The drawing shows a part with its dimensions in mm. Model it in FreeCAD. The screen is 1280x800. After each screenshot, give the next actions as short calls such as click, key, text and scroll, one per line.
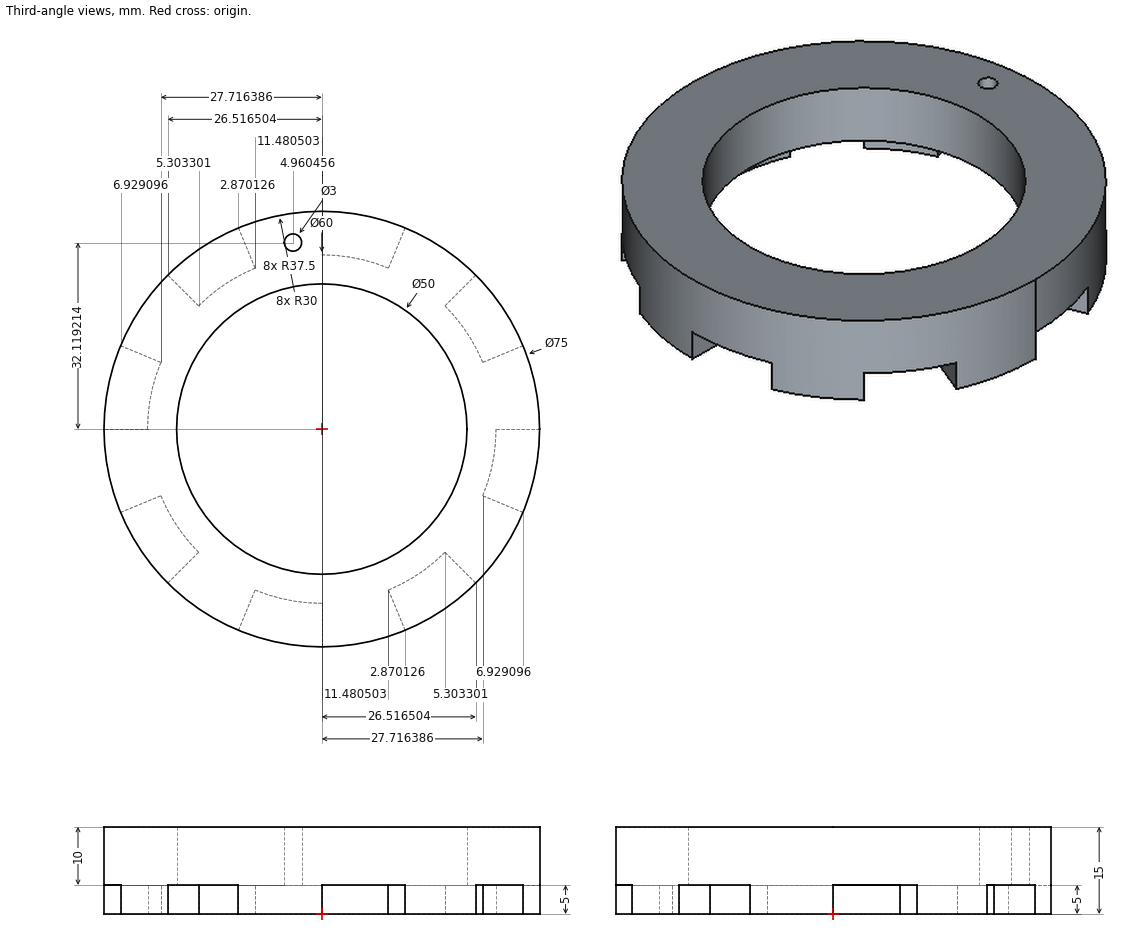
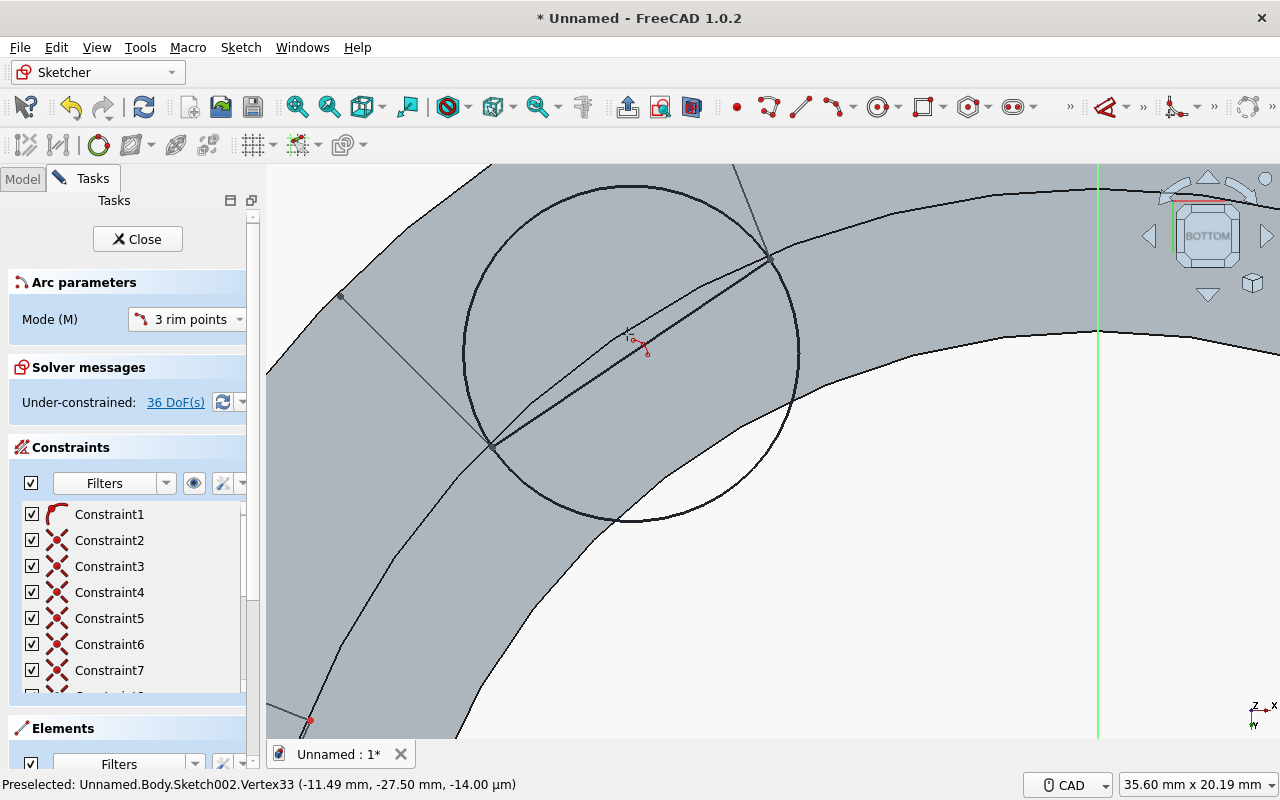
click(623, 333)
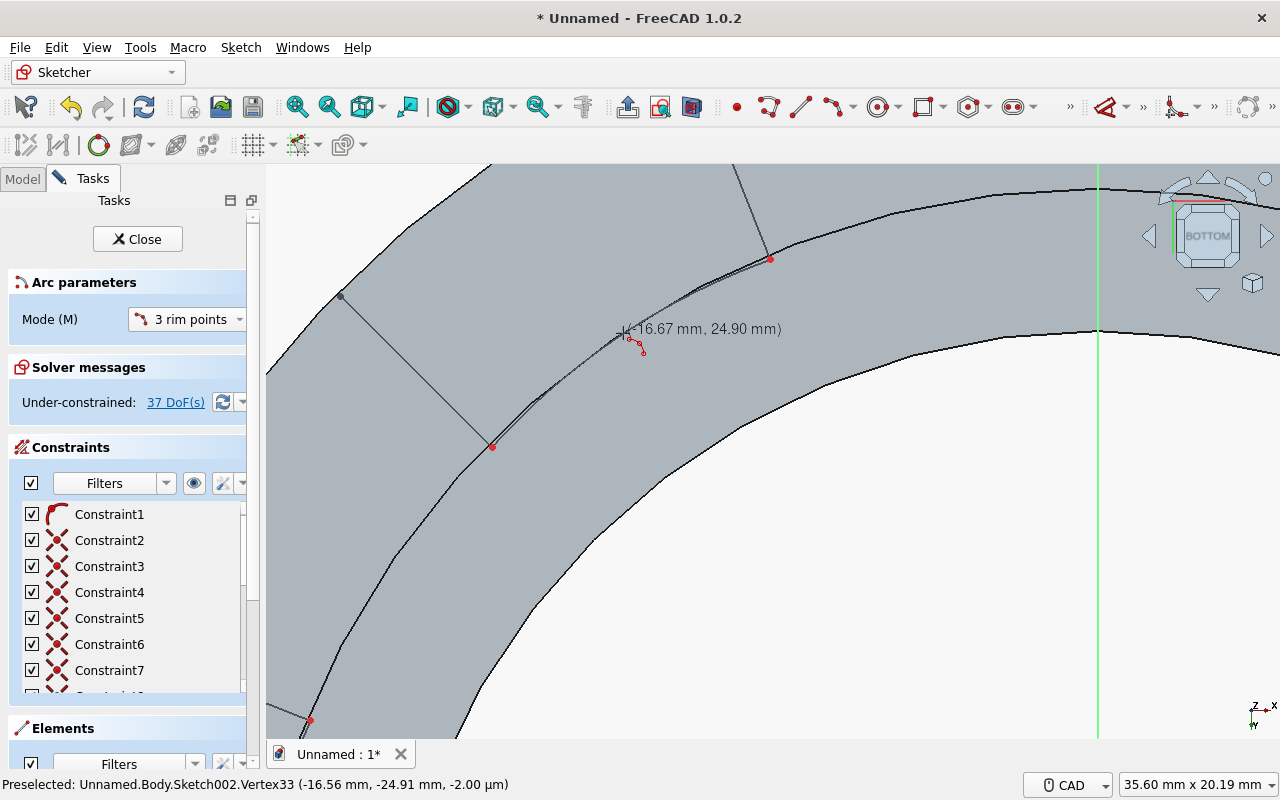
scroll(627, 334, down, 9)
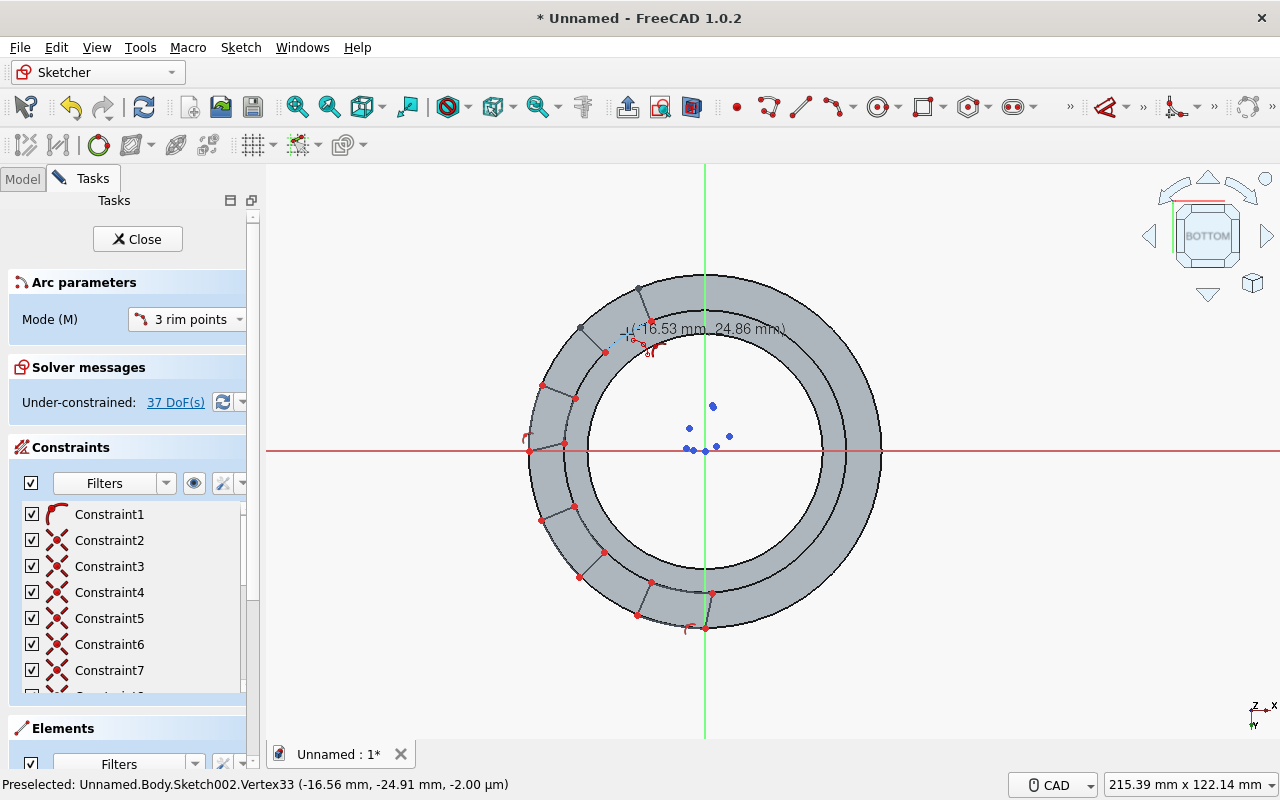
click(638, 289)
click(580, 328)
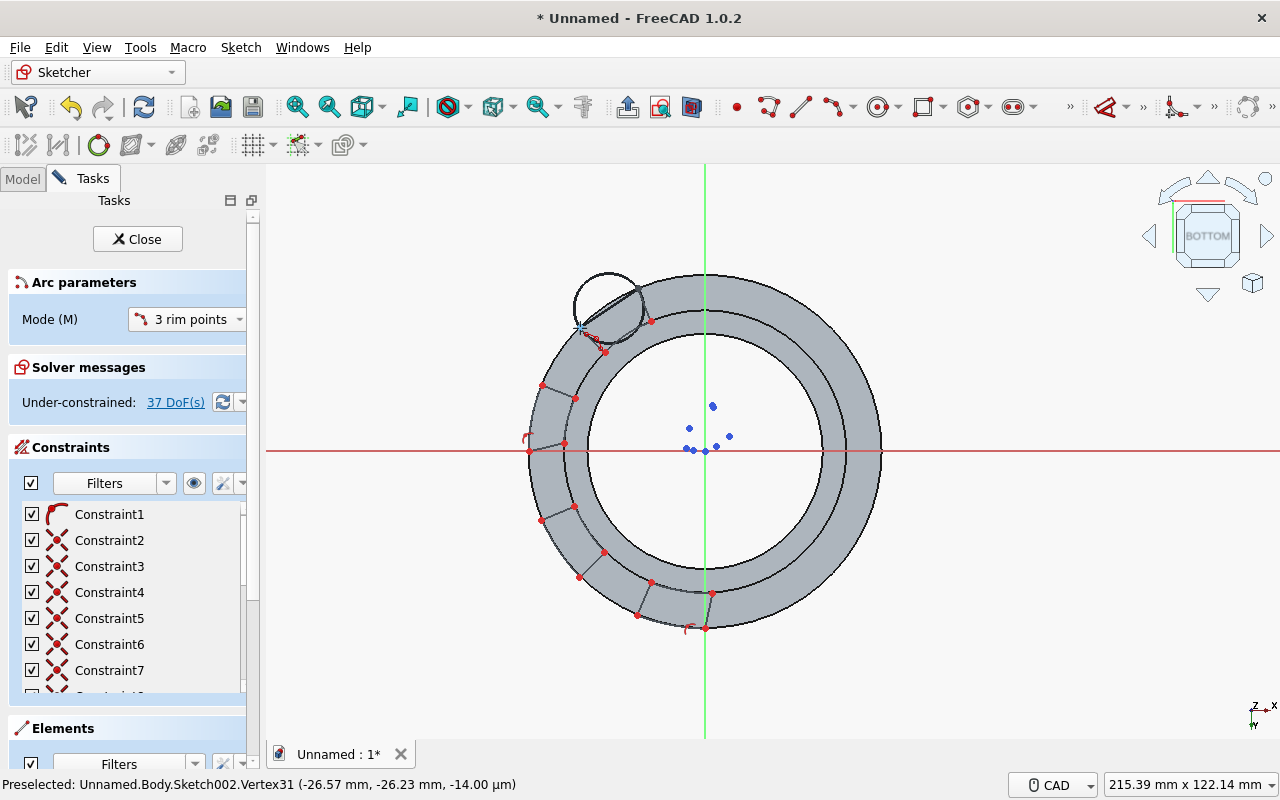
scroll(607, 305, up, 8)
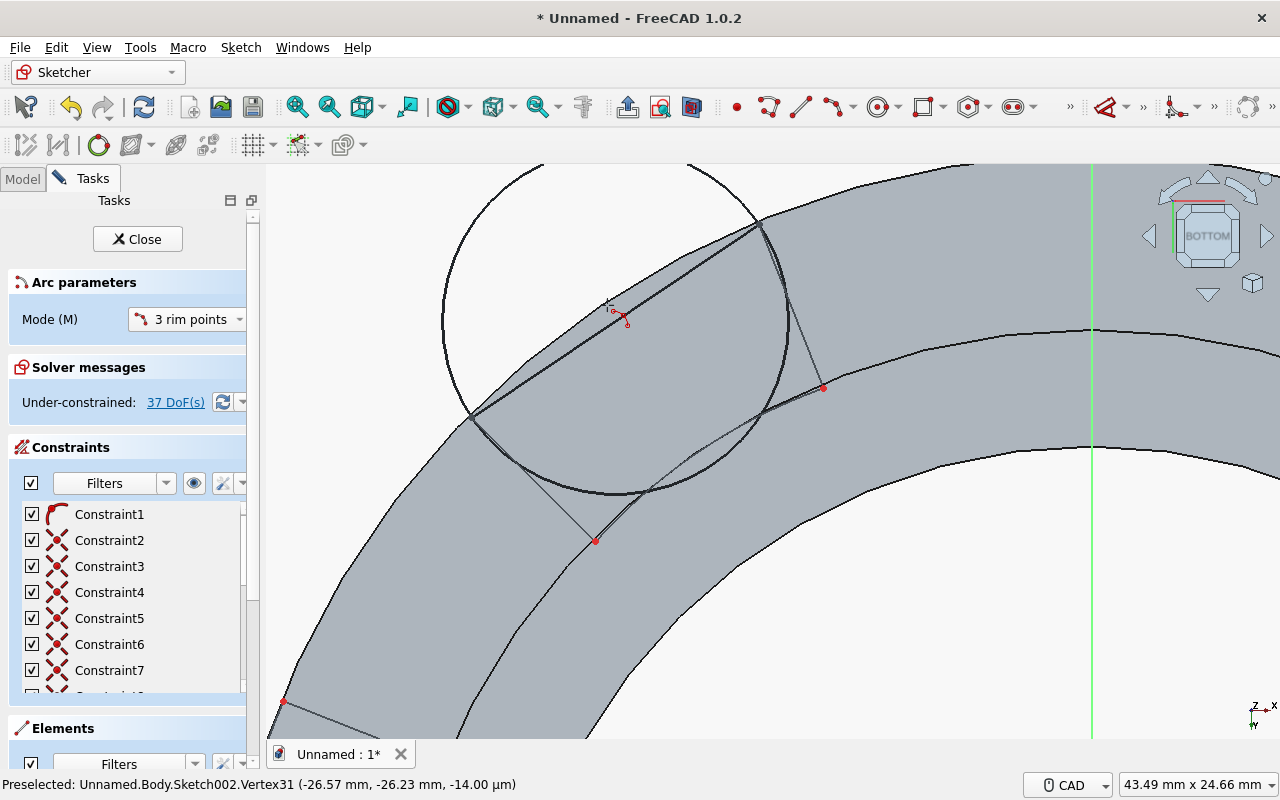
click(606, 302)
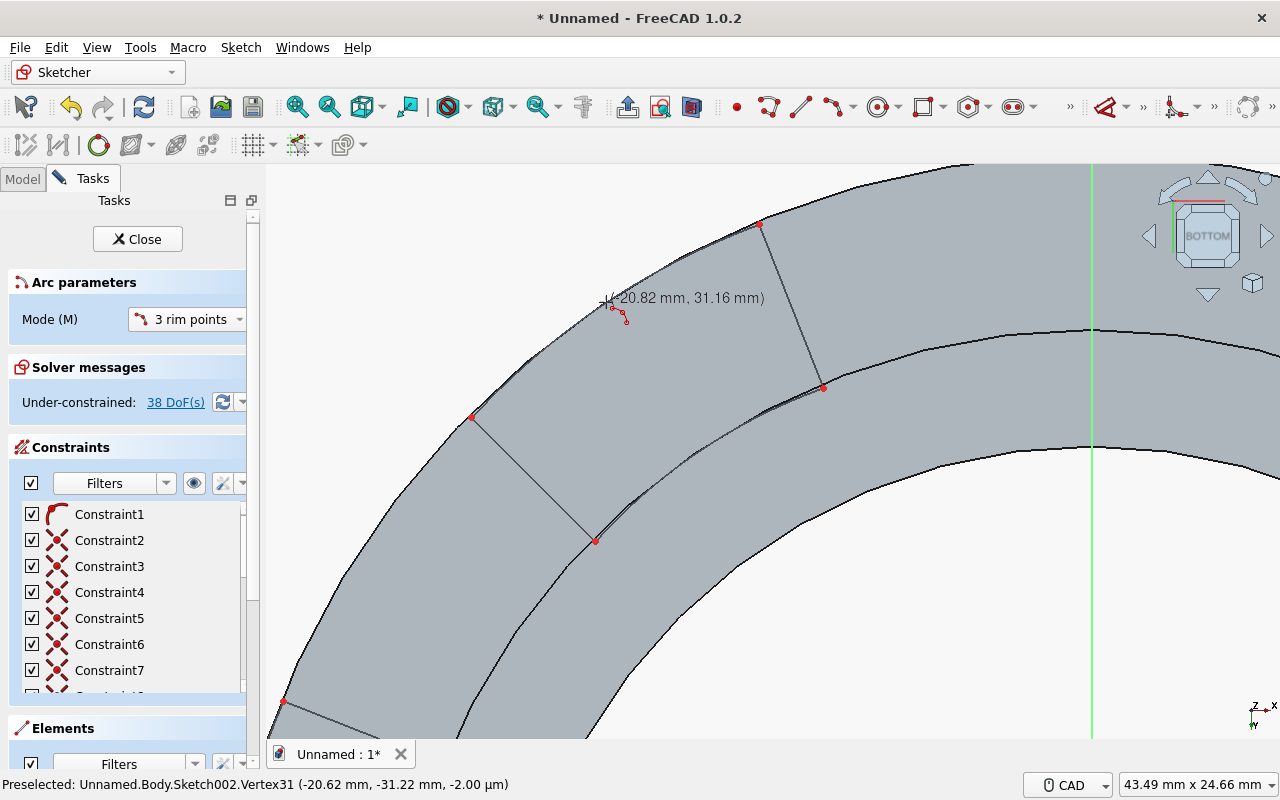
click(802, 108)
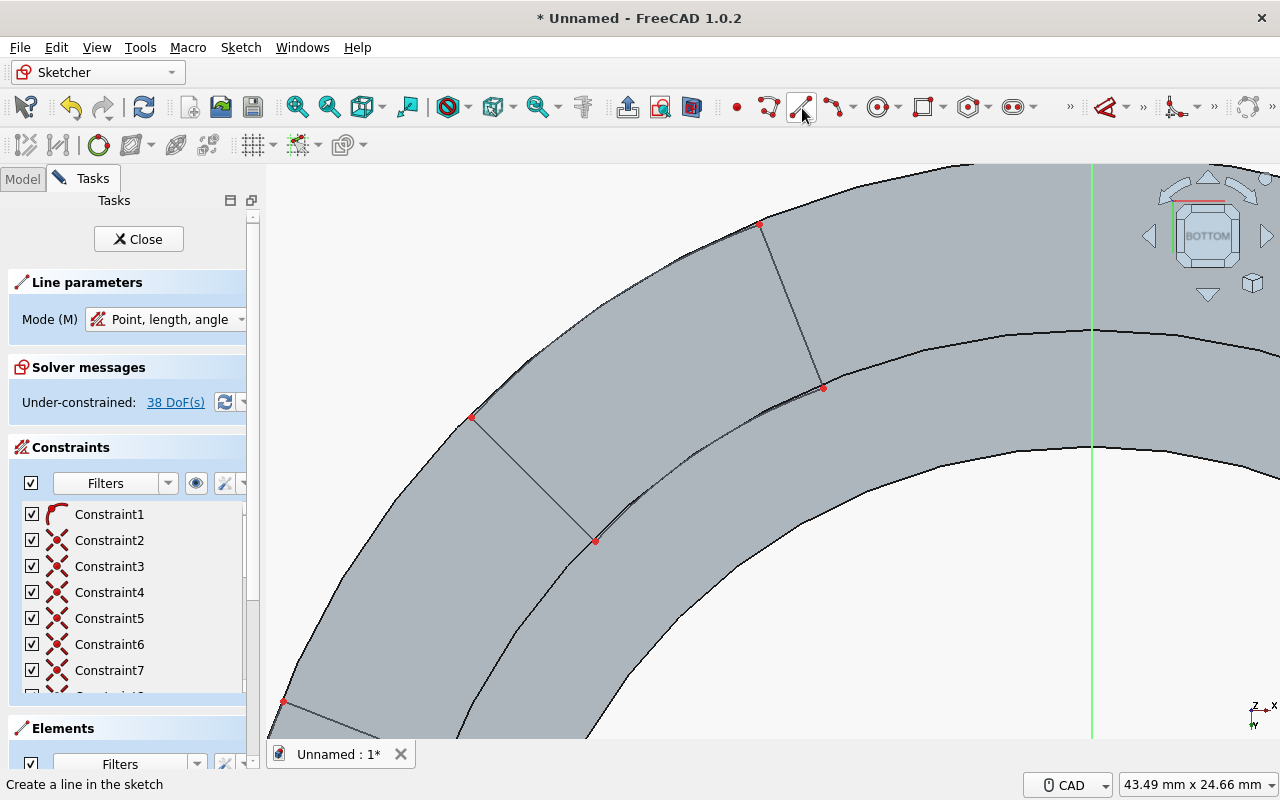
scroll(607, 305, down, 8)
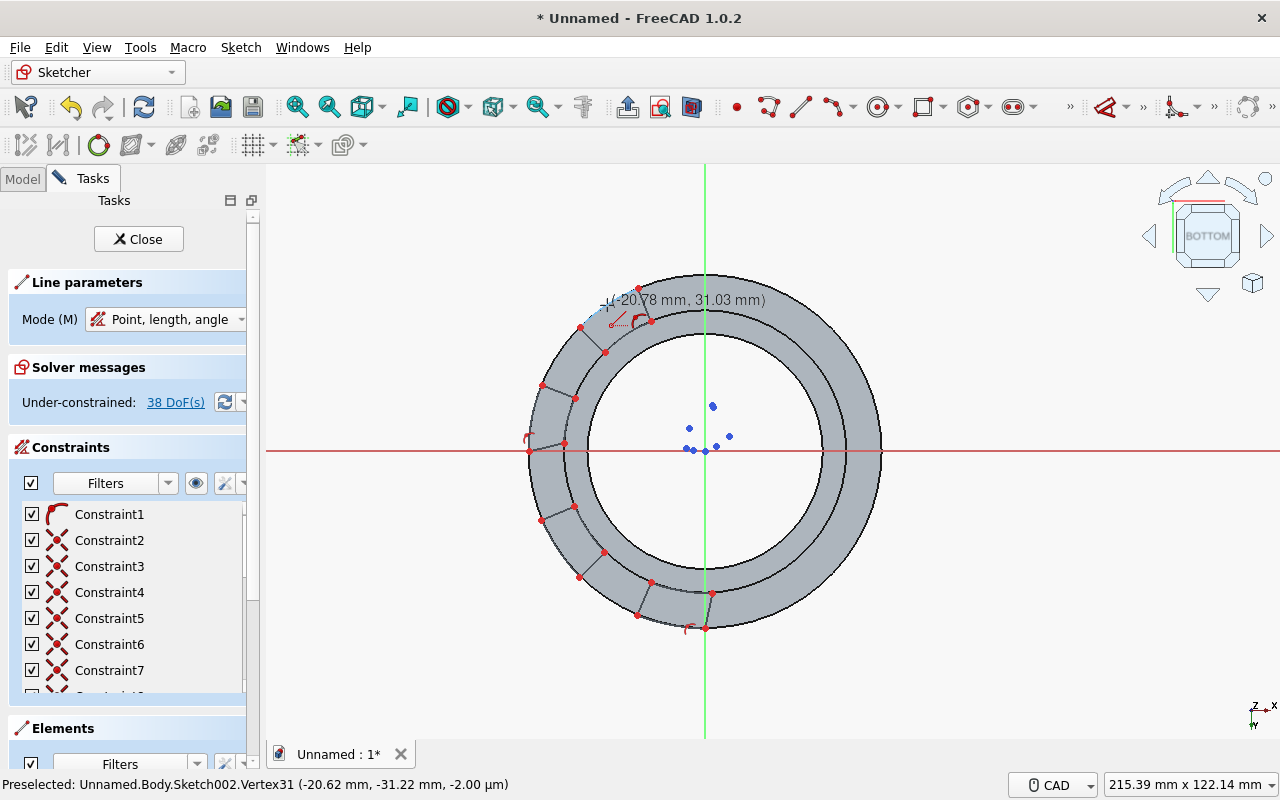
click(705, 275)
click(714, 310)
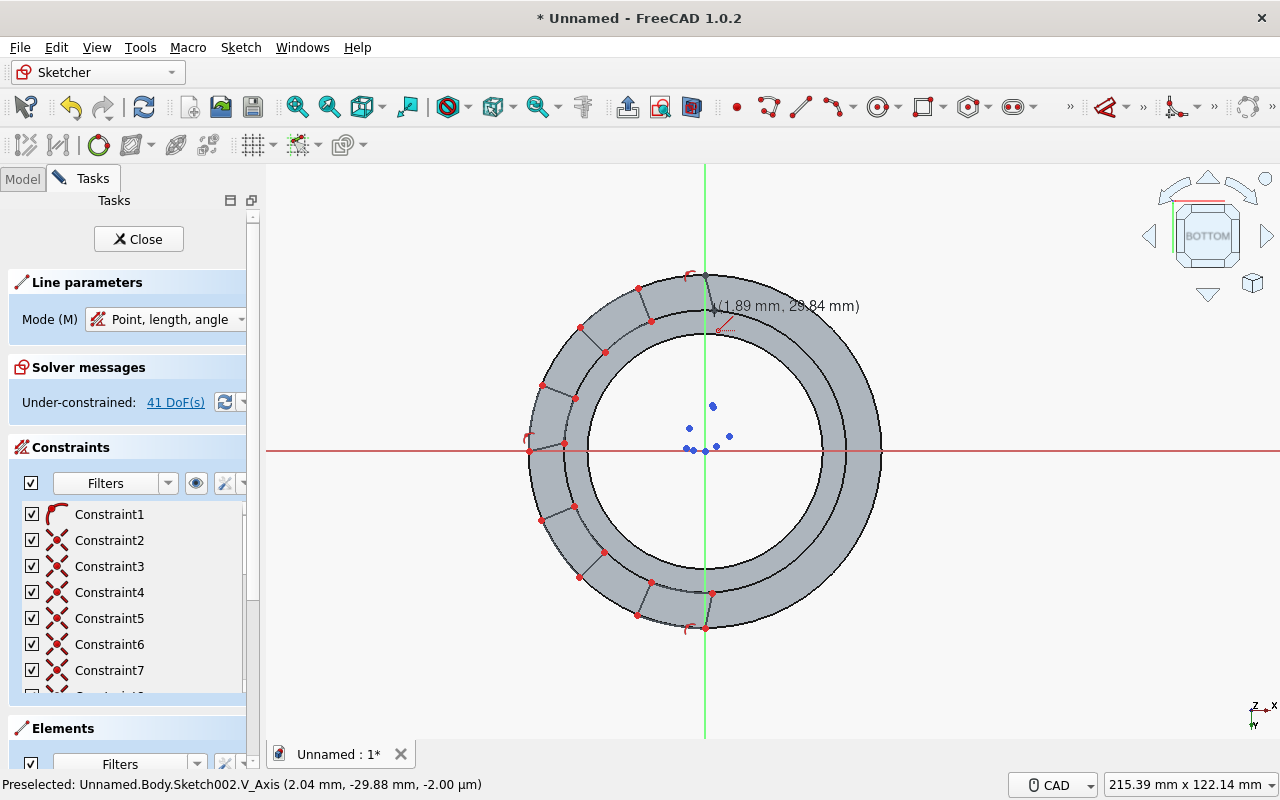
click(759, 321)
click(773, 288)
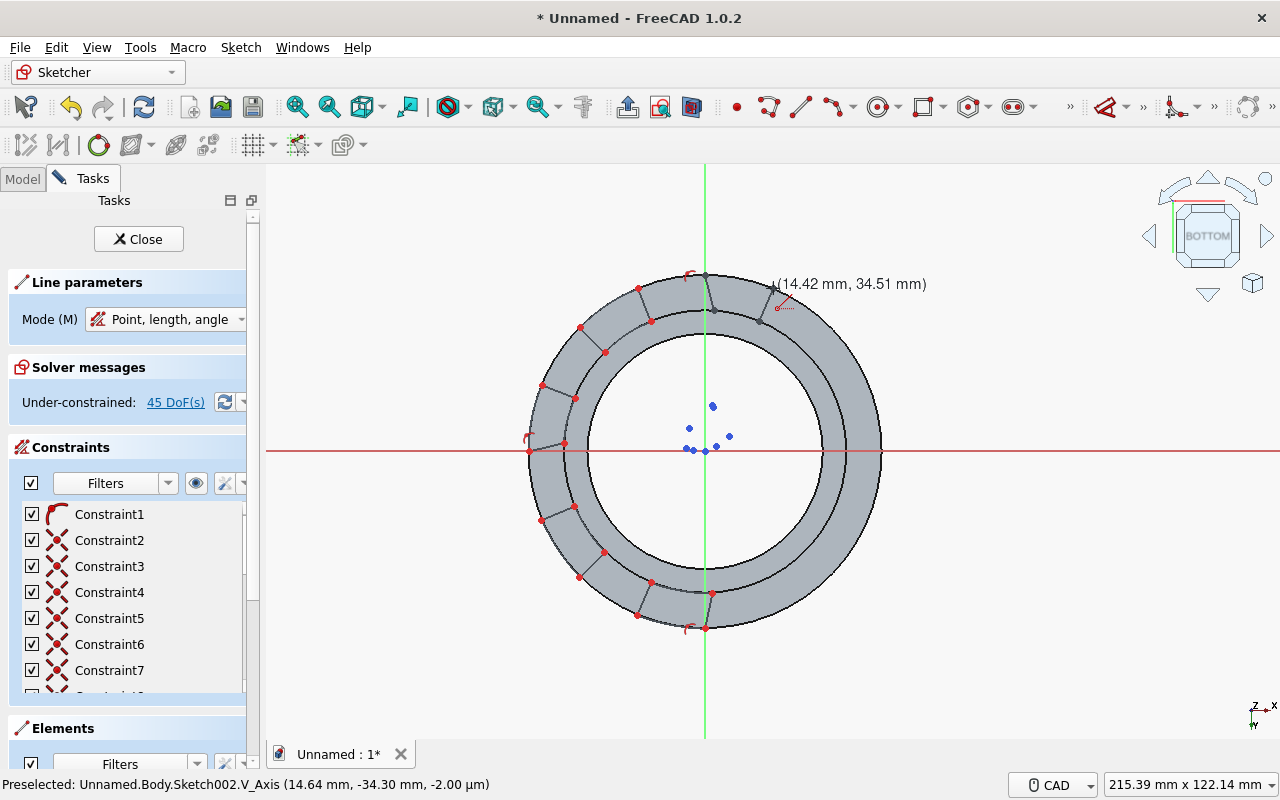
key(g)
key(3)
key(a)